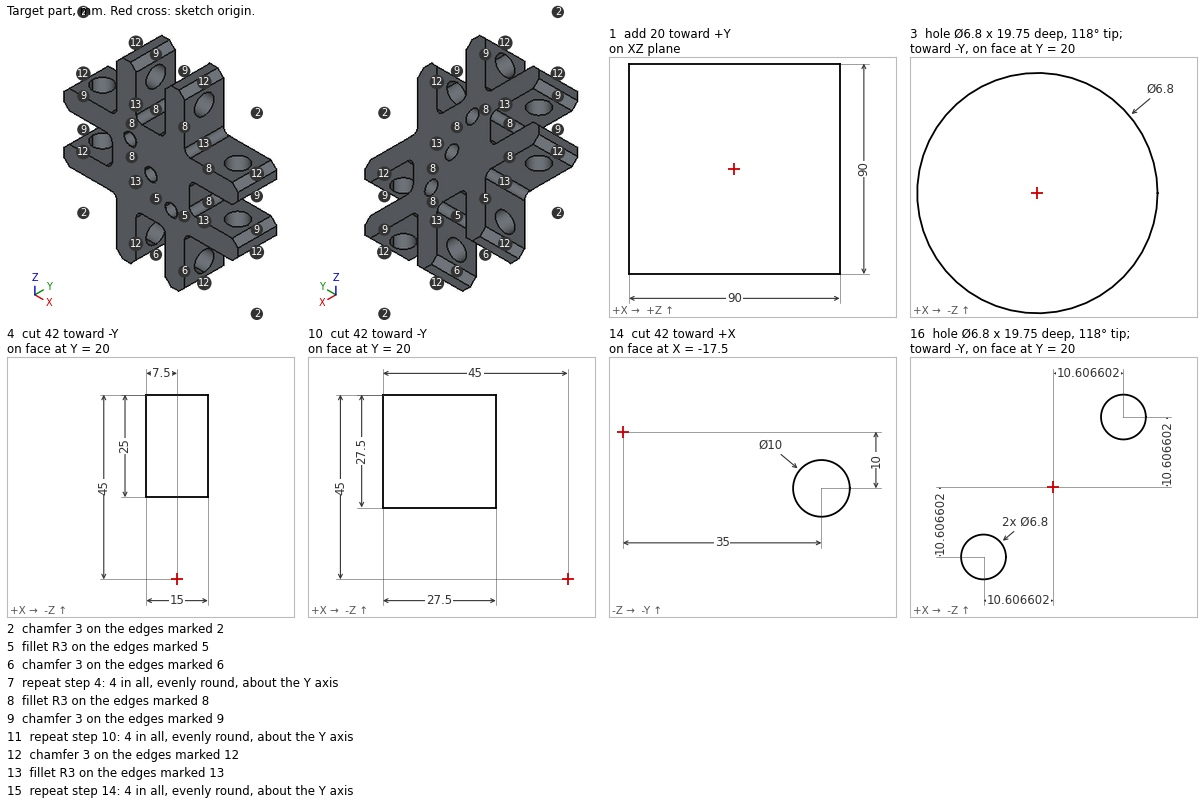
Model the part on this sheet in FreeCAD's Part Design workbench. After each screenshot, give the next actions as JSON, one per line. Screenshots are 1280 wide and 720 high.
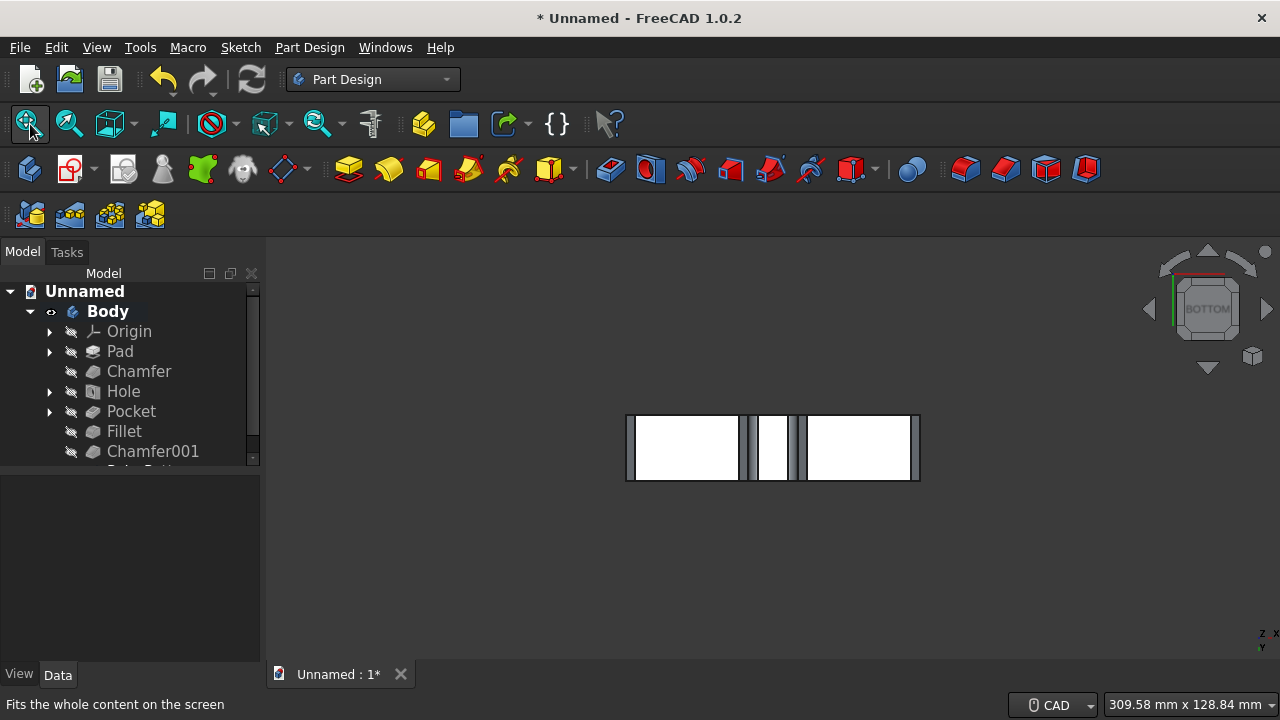
{"action": "key", "text": "0"}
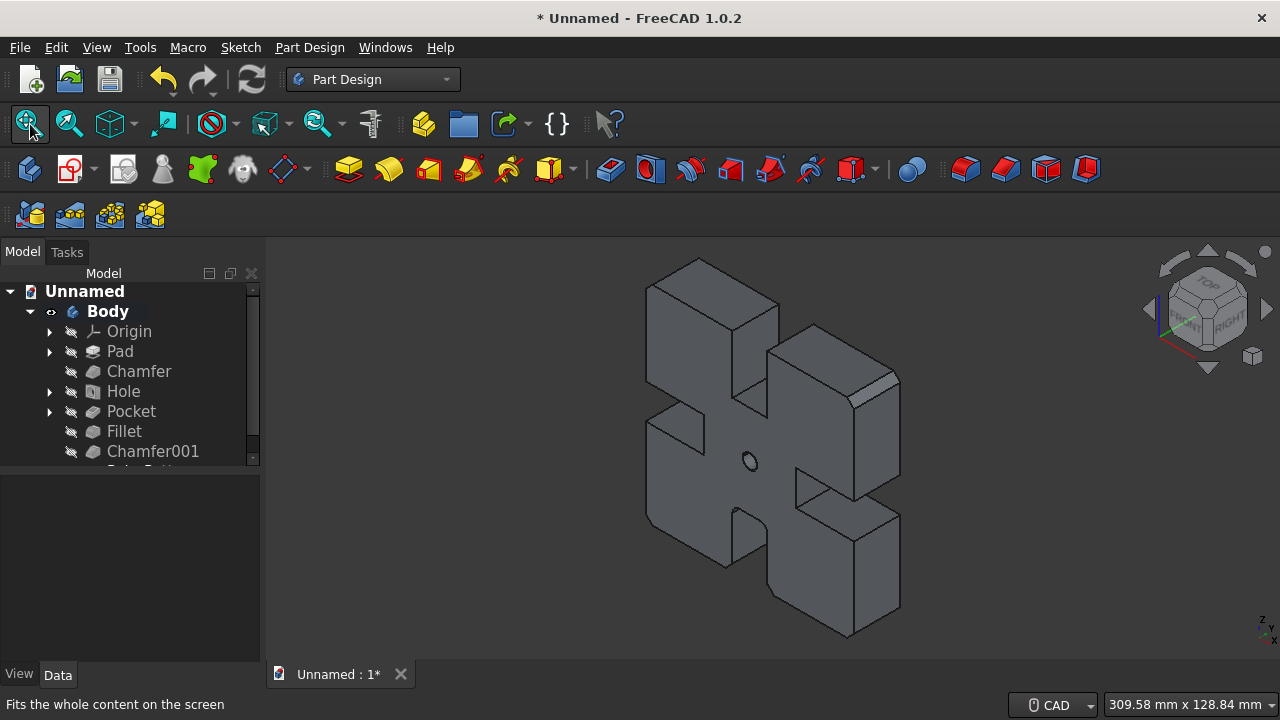
{"action": "key", "text": "2"}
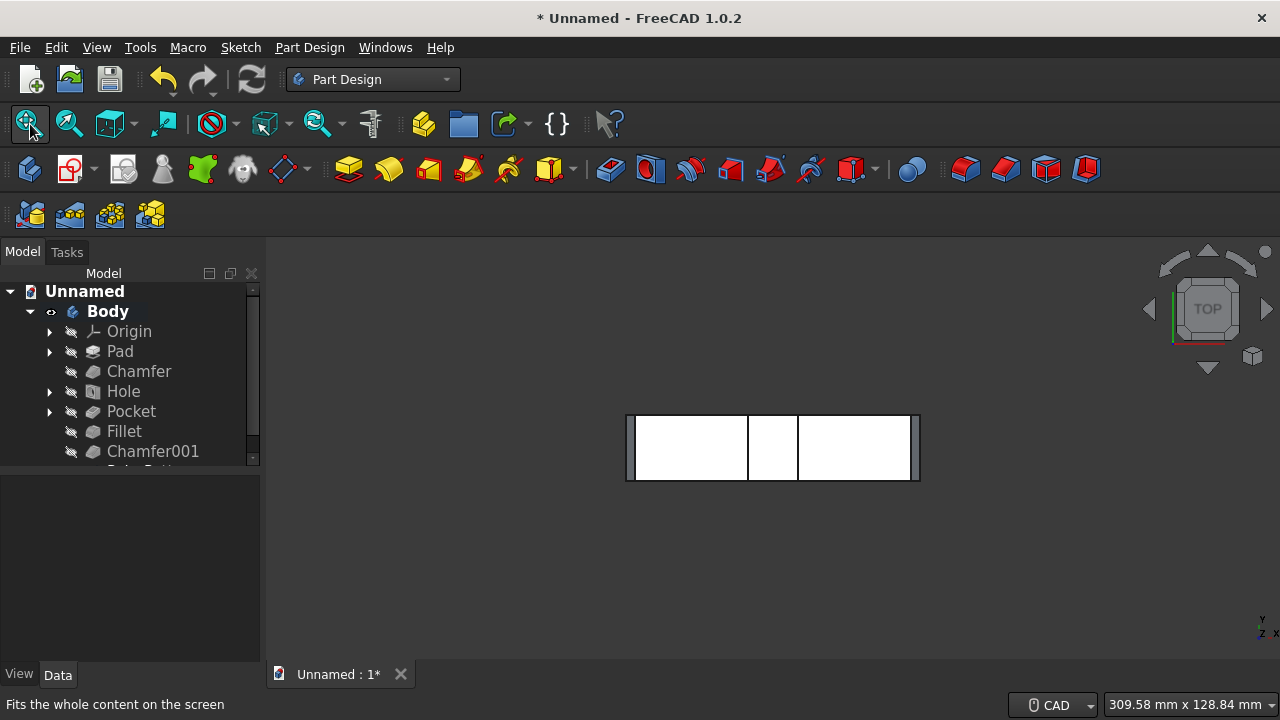
{"action": "left_click", "coordinate": [30, 124]}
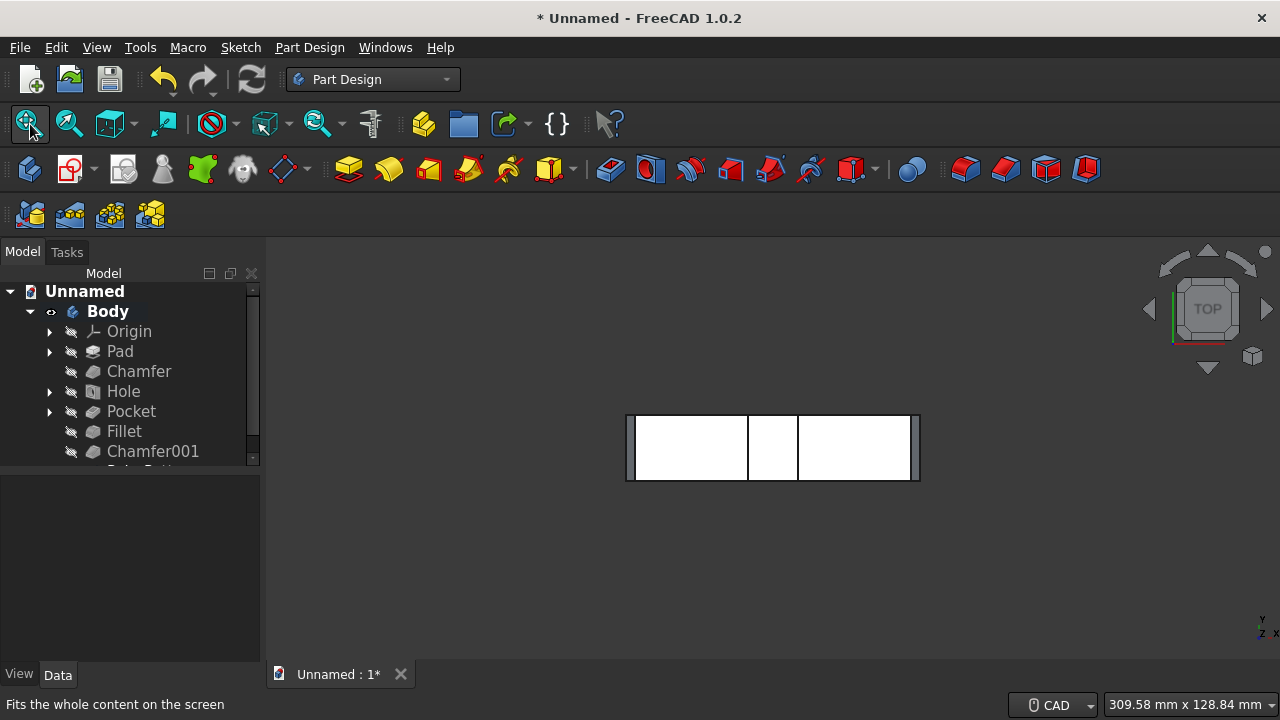
{"action": "key", "text": "1"}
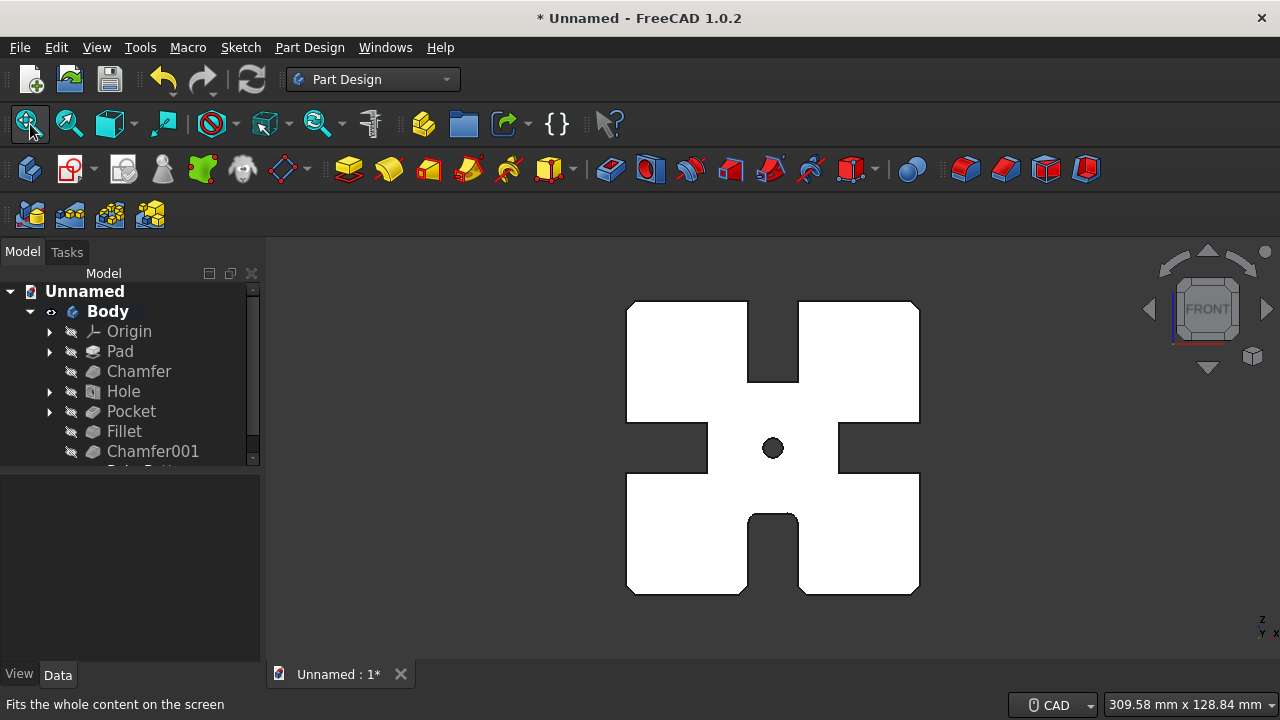
{"action": "key", "text": "3"}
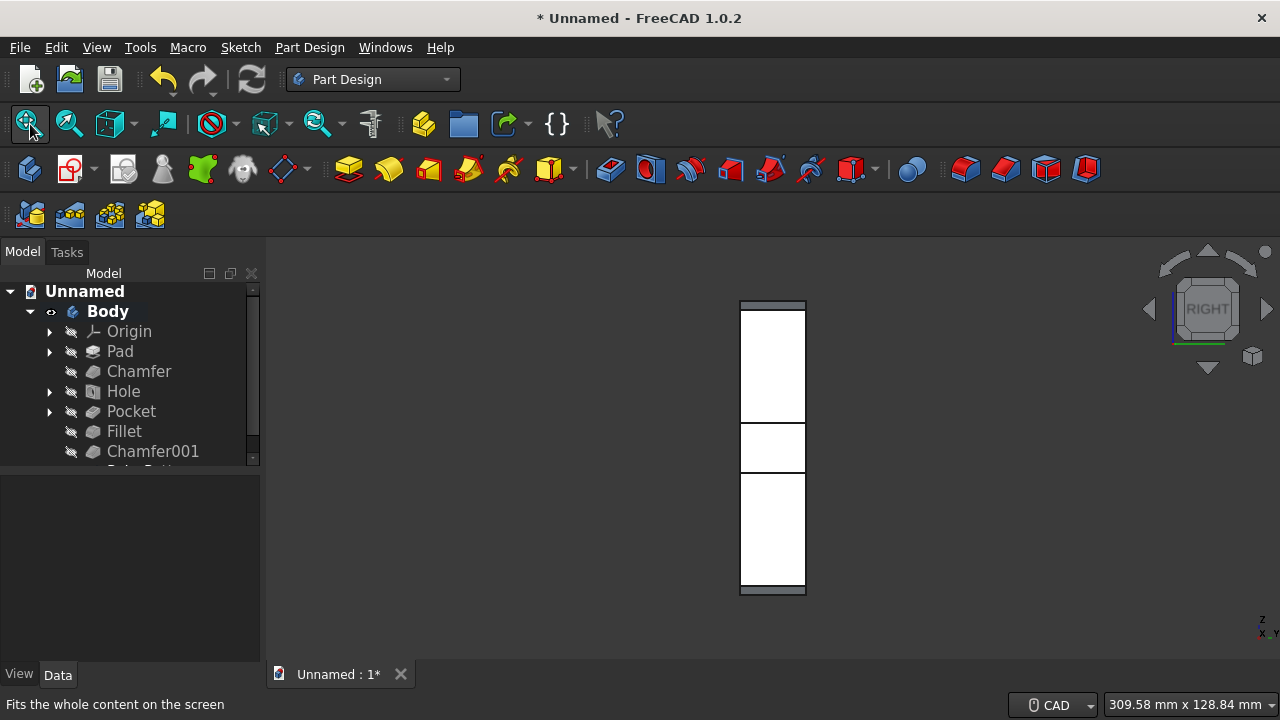
{"action": "key", "text": "5"}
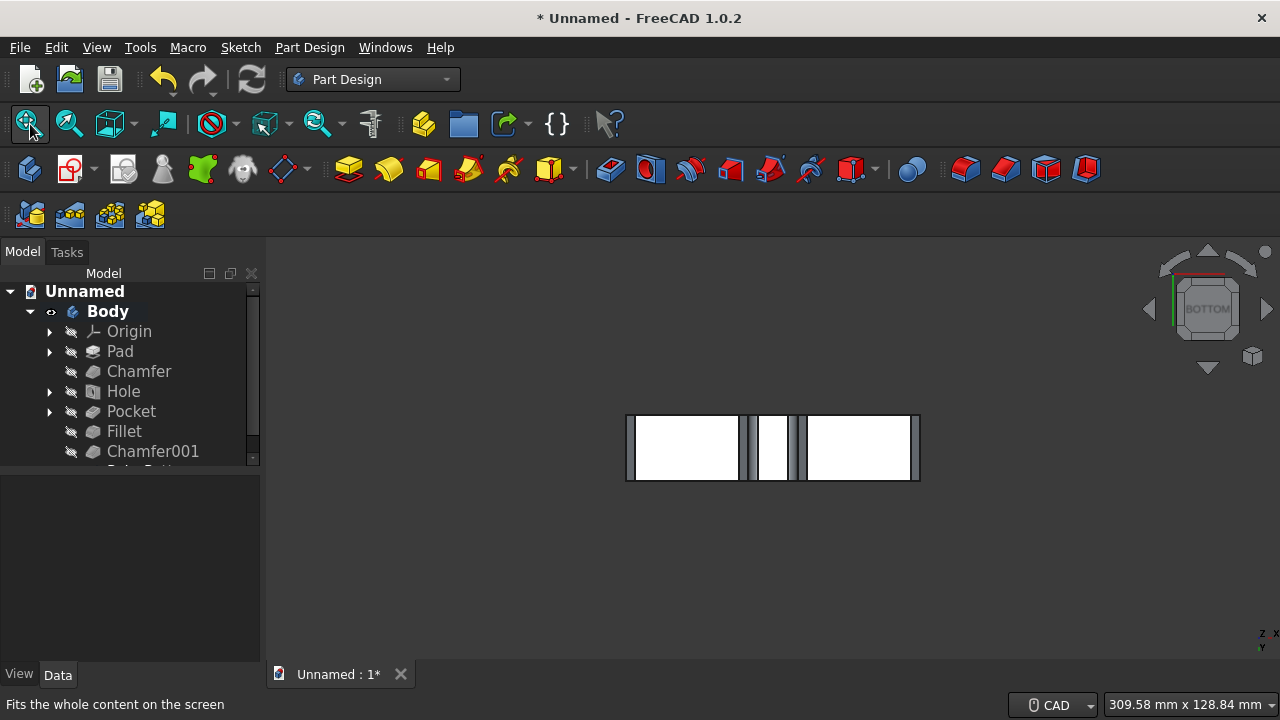
{"action": "left_click", "coordinate": [30, 124]}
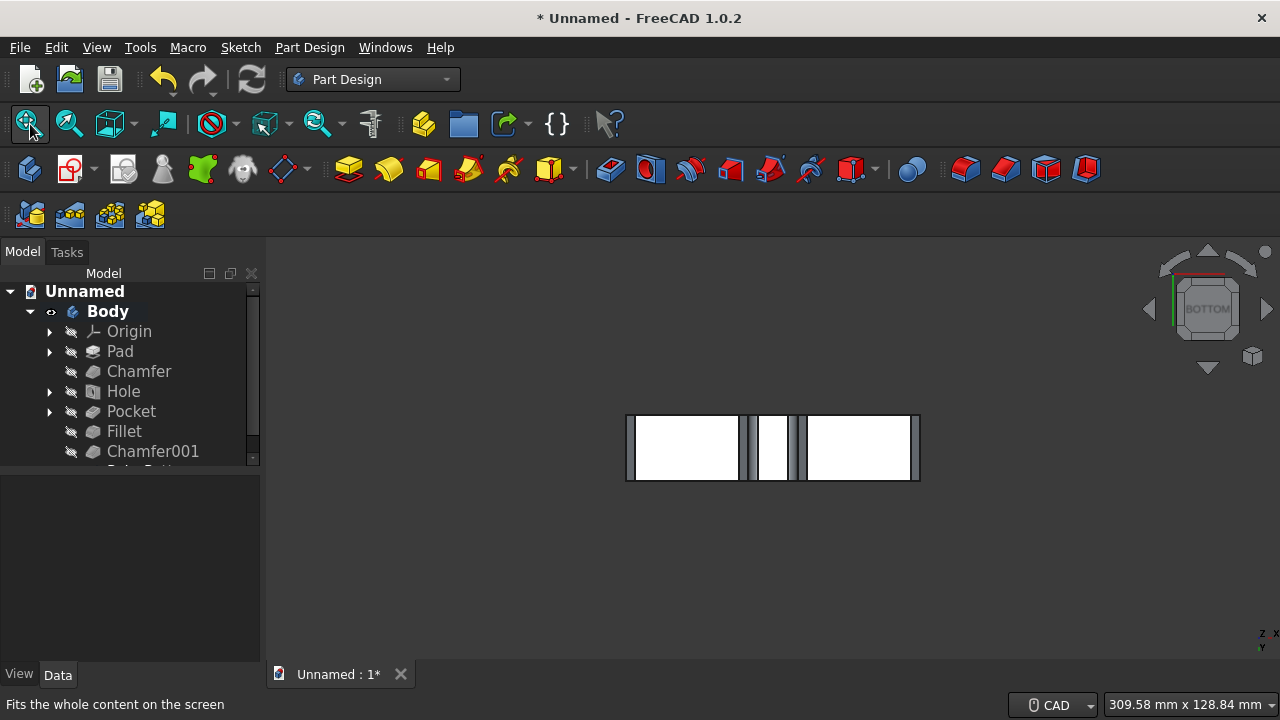
{"action": "key", "text": "4"}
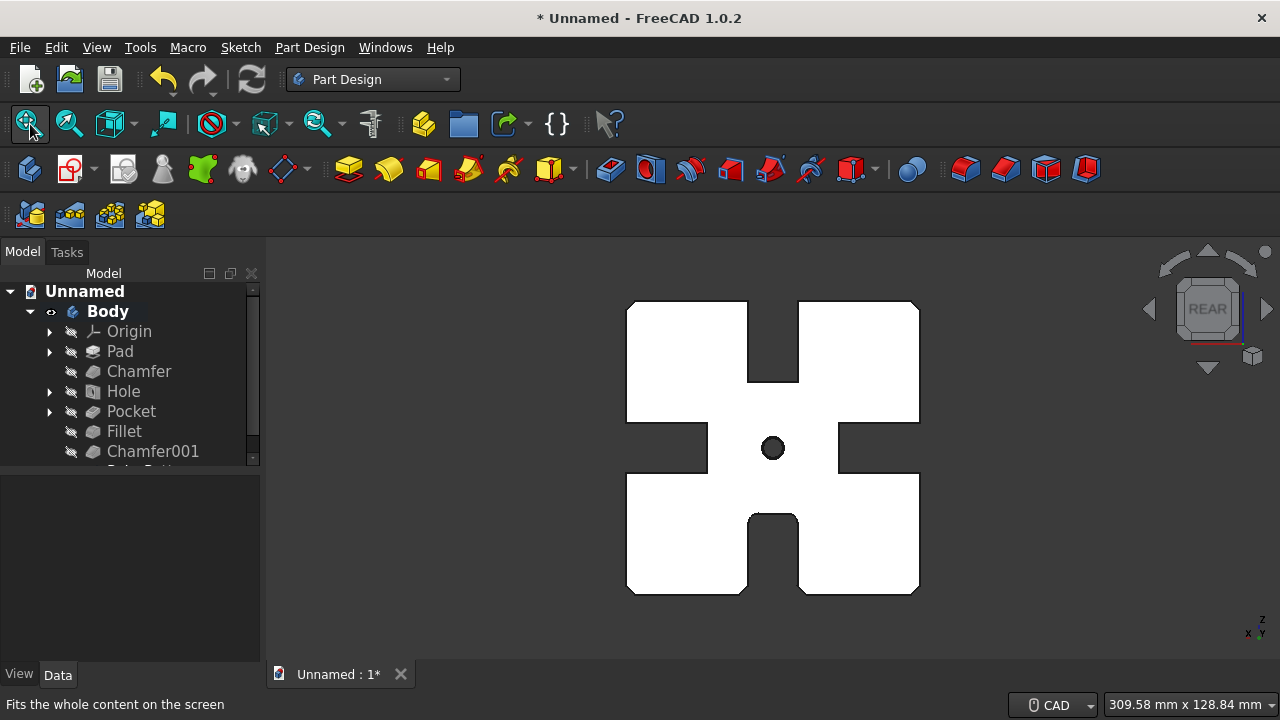
{"action": "key", "text": "6"}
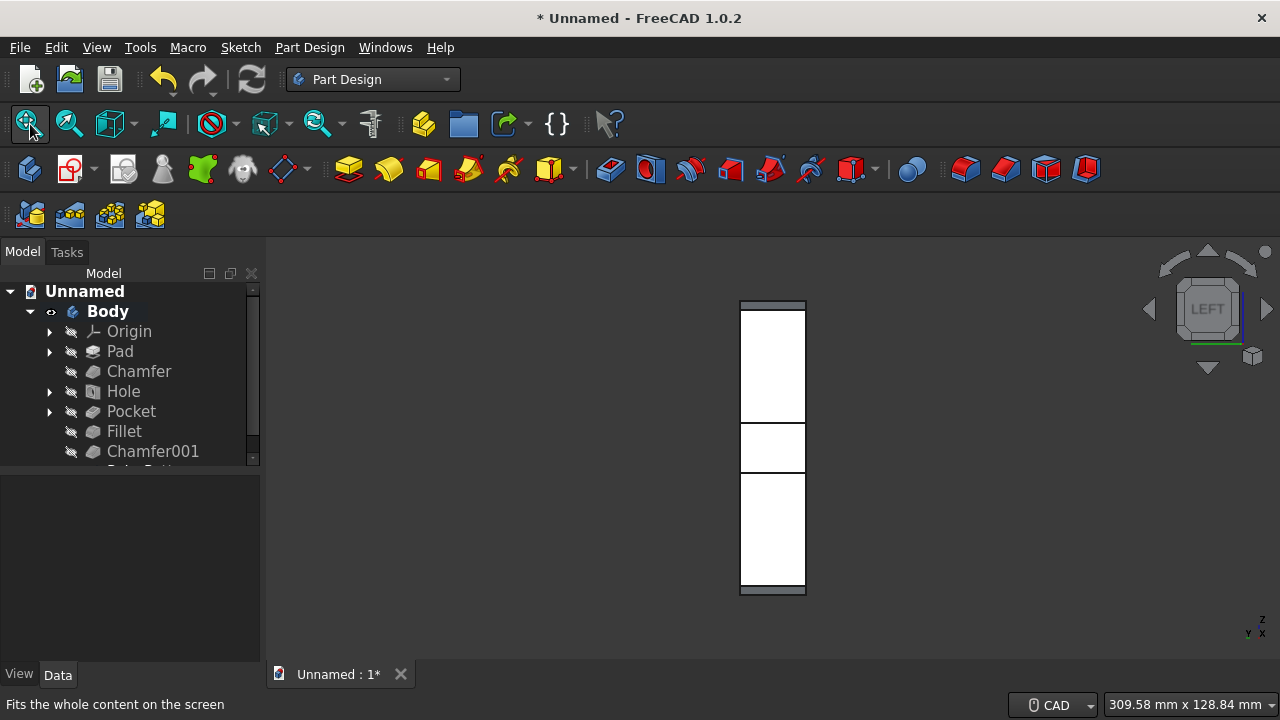
{"action": "key", "text": "v 3"}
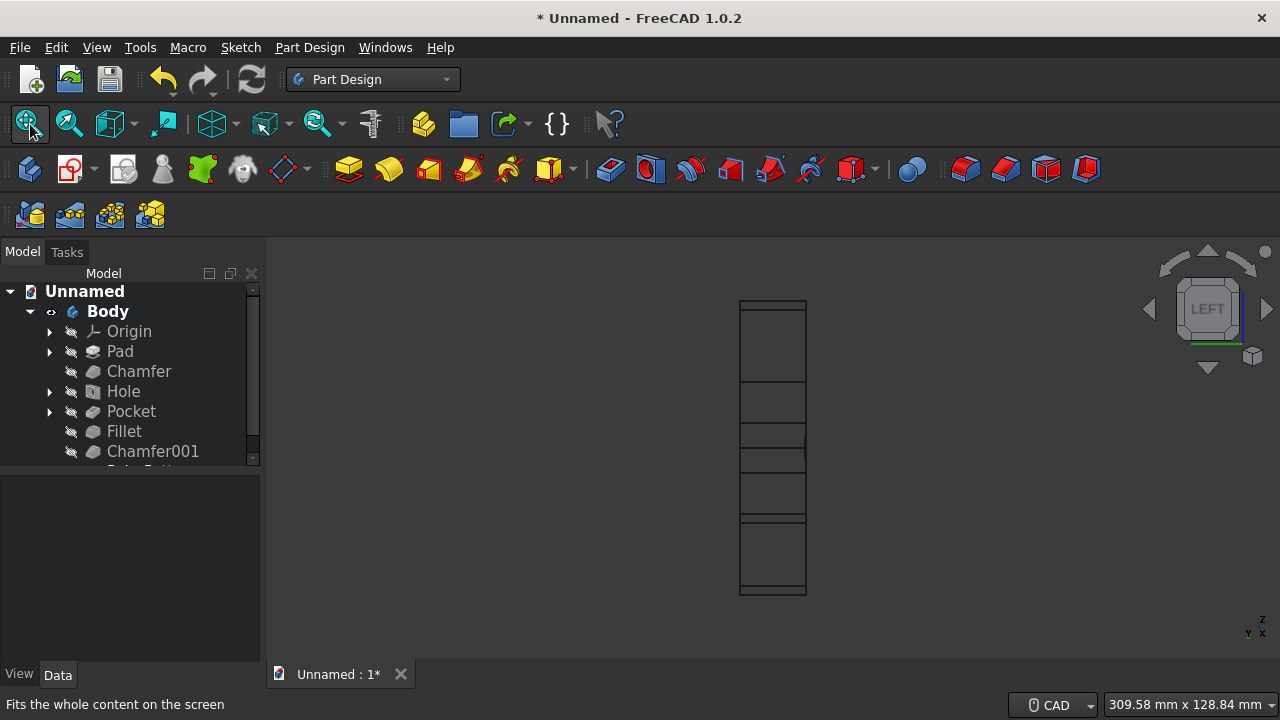
{"action": "key", "text": "0"}